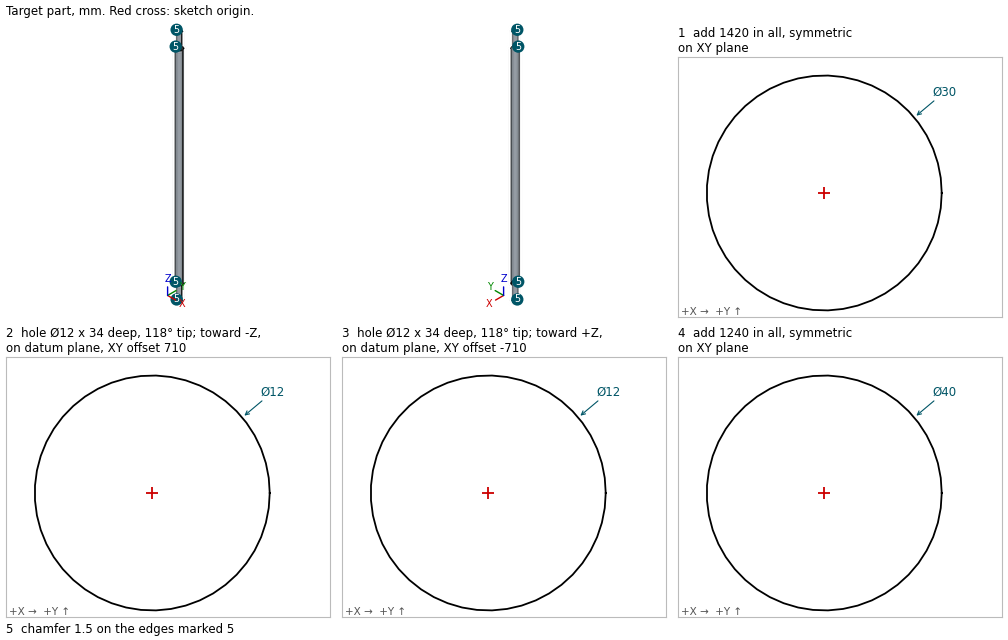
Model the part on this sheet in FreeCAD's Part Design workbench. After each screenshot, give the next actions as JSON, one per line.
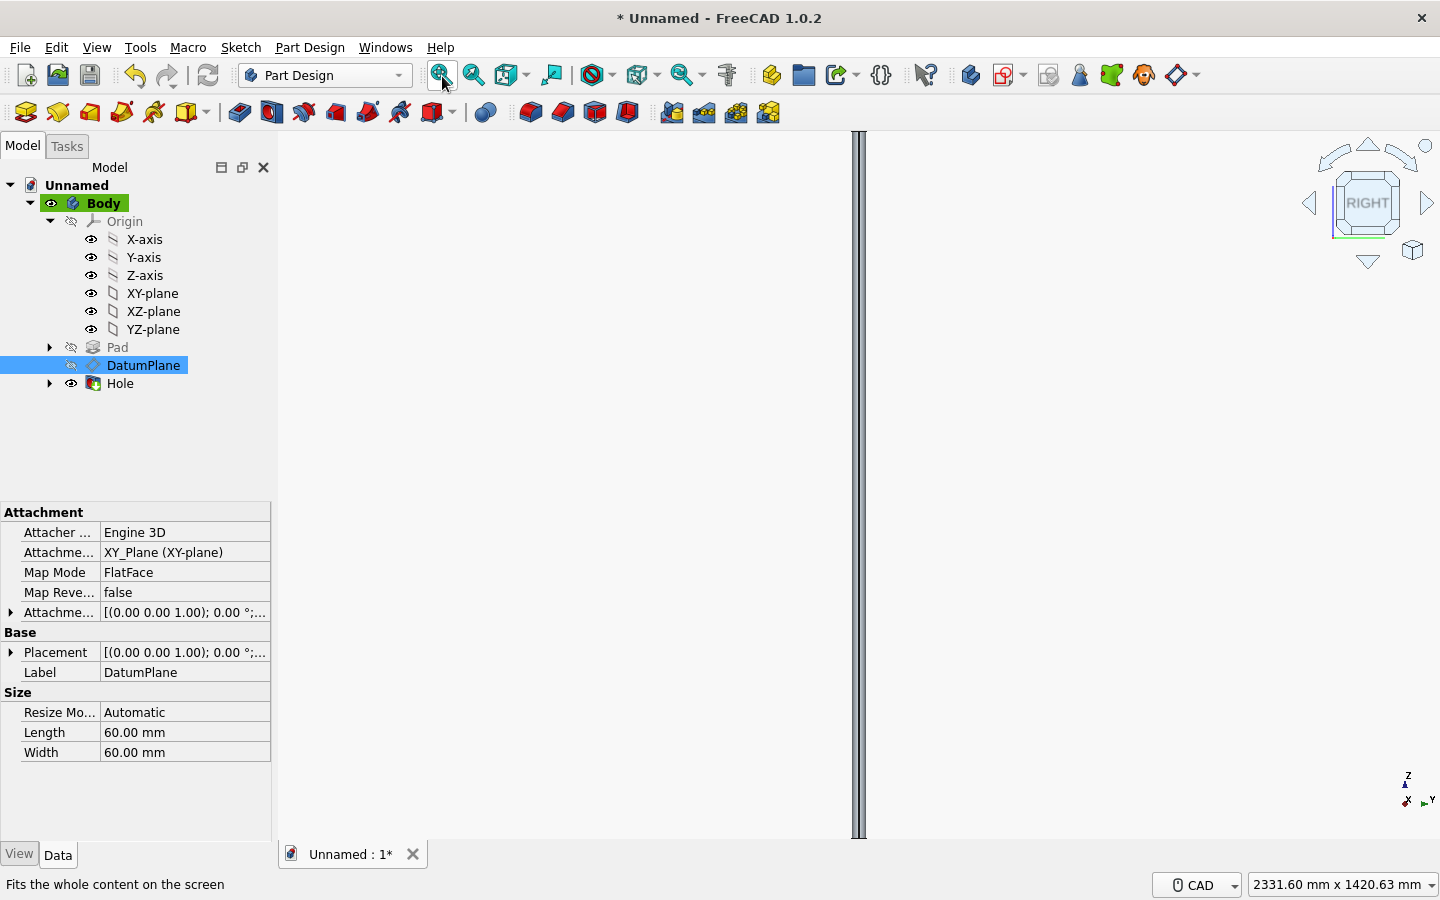
{"action": "left_click", "coordinate": [136, 293]}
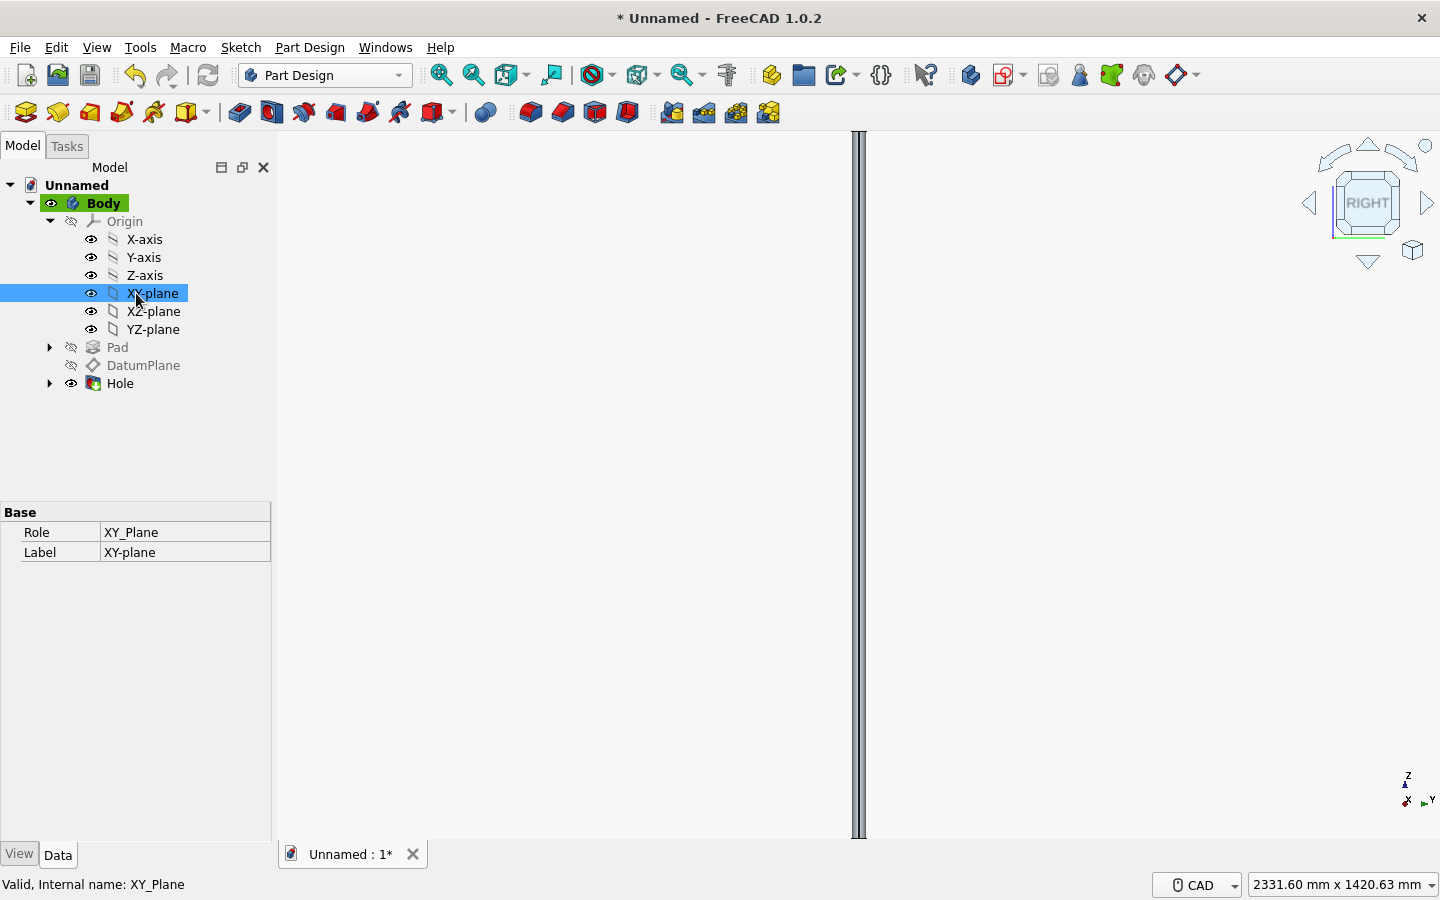
{"action": "left_click", "coordinate": [1176, 76]}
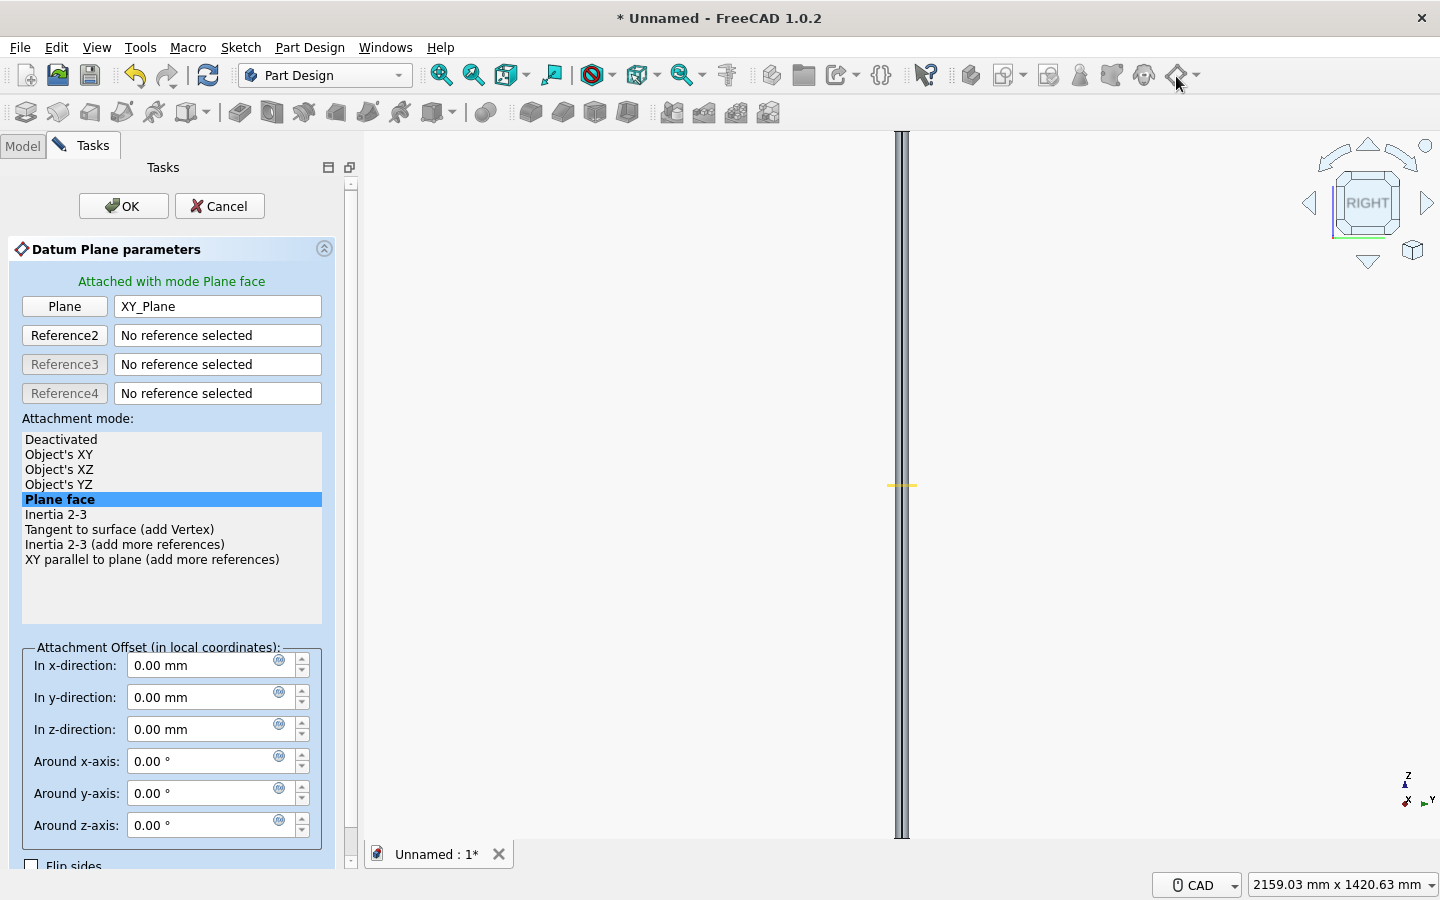
{"action": "triple_click", "coordinate": [210, 729]}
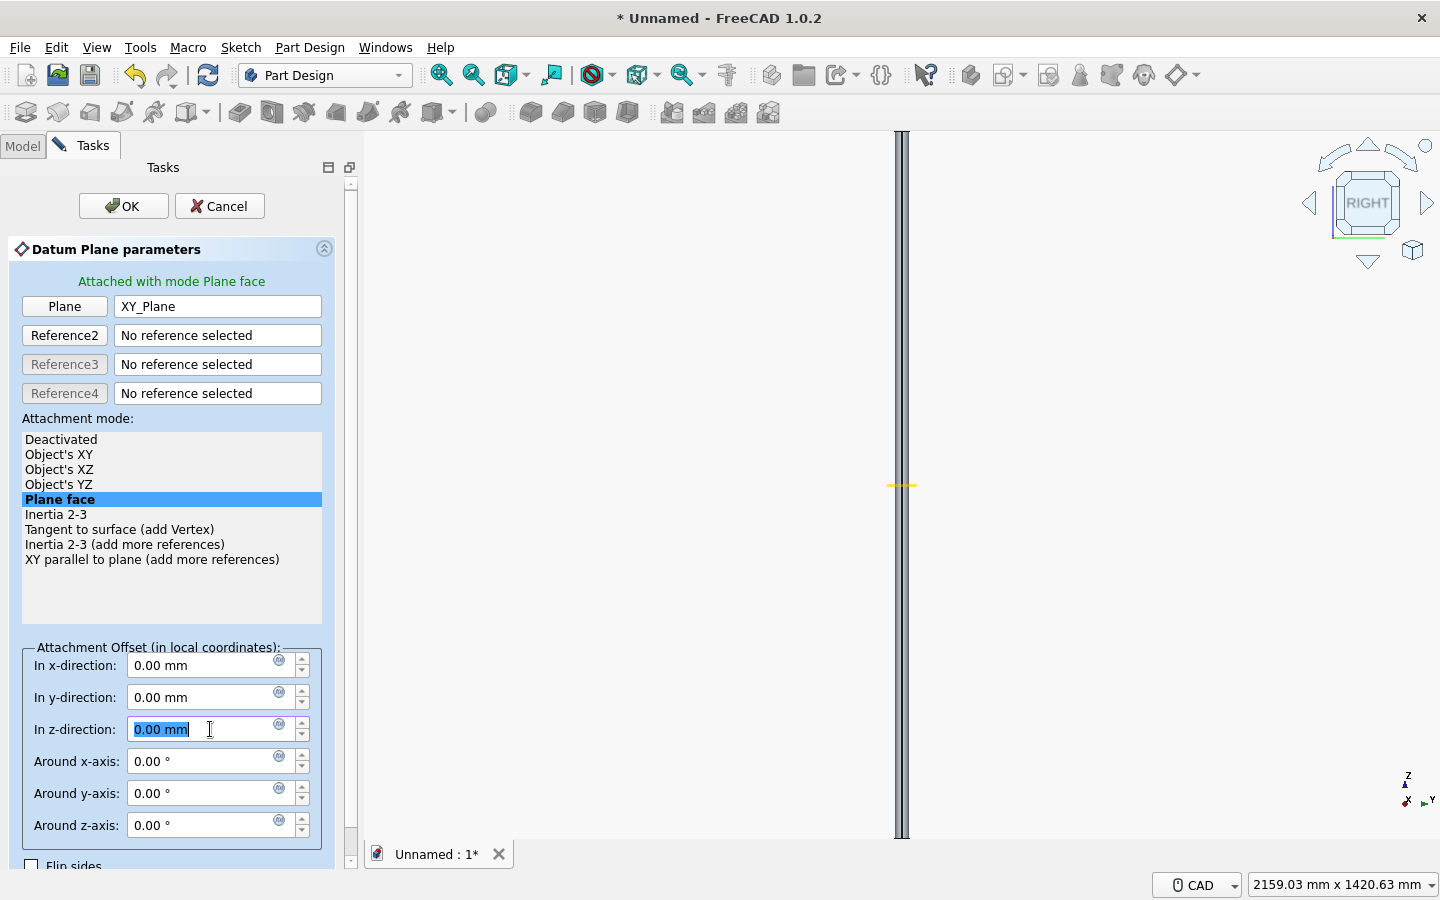
{"action": "type", "text": "-710"}
{"action": "key", "text": "Tab"}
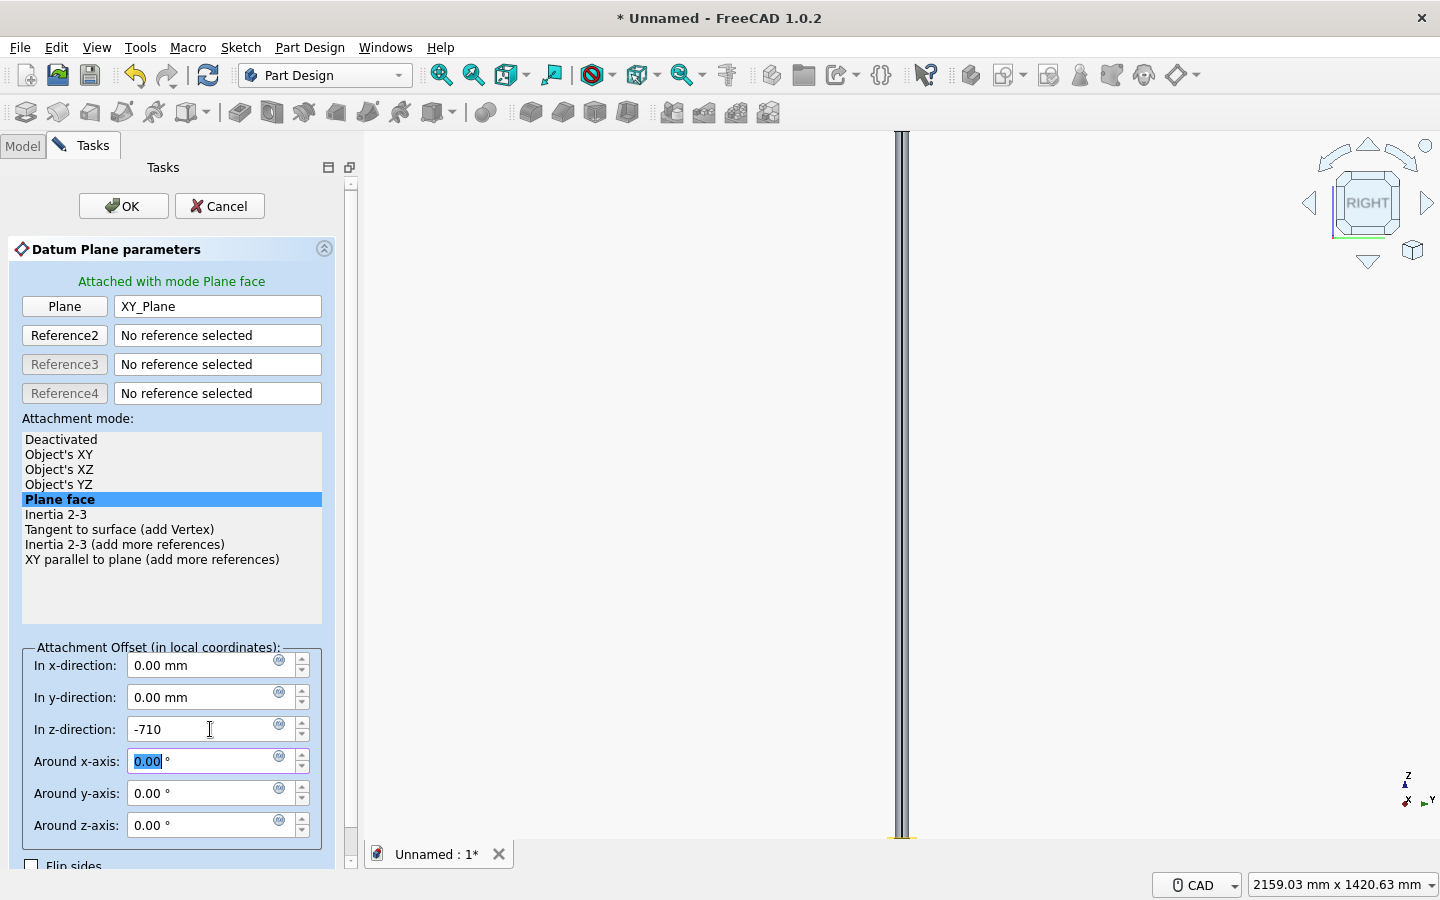
{"action": "left_click", "coordinate": [124, 206]}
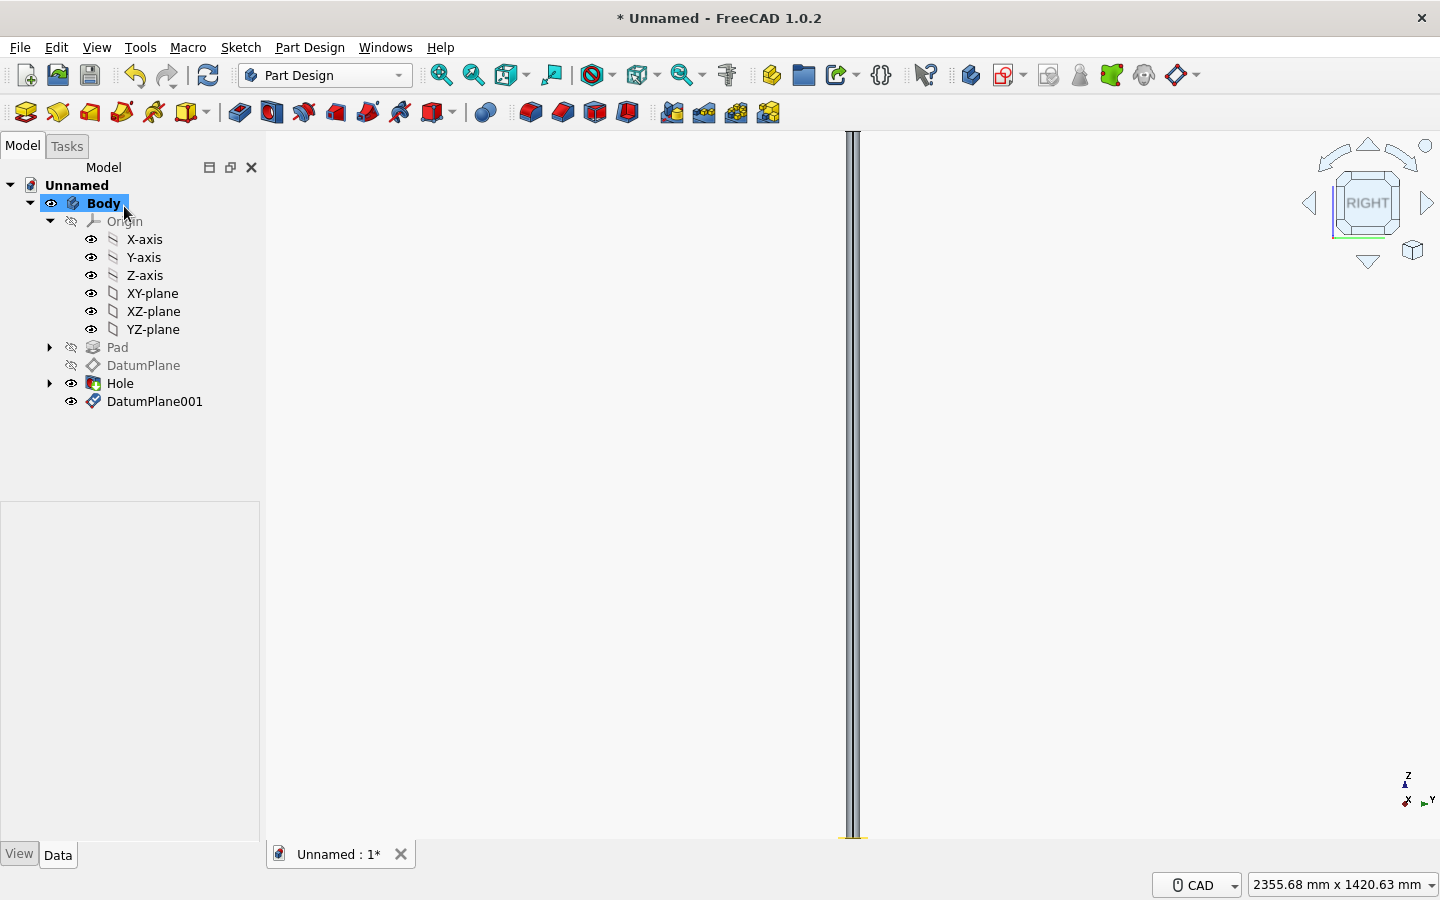
{"action": "left_click", "coordinate": [116, 401]}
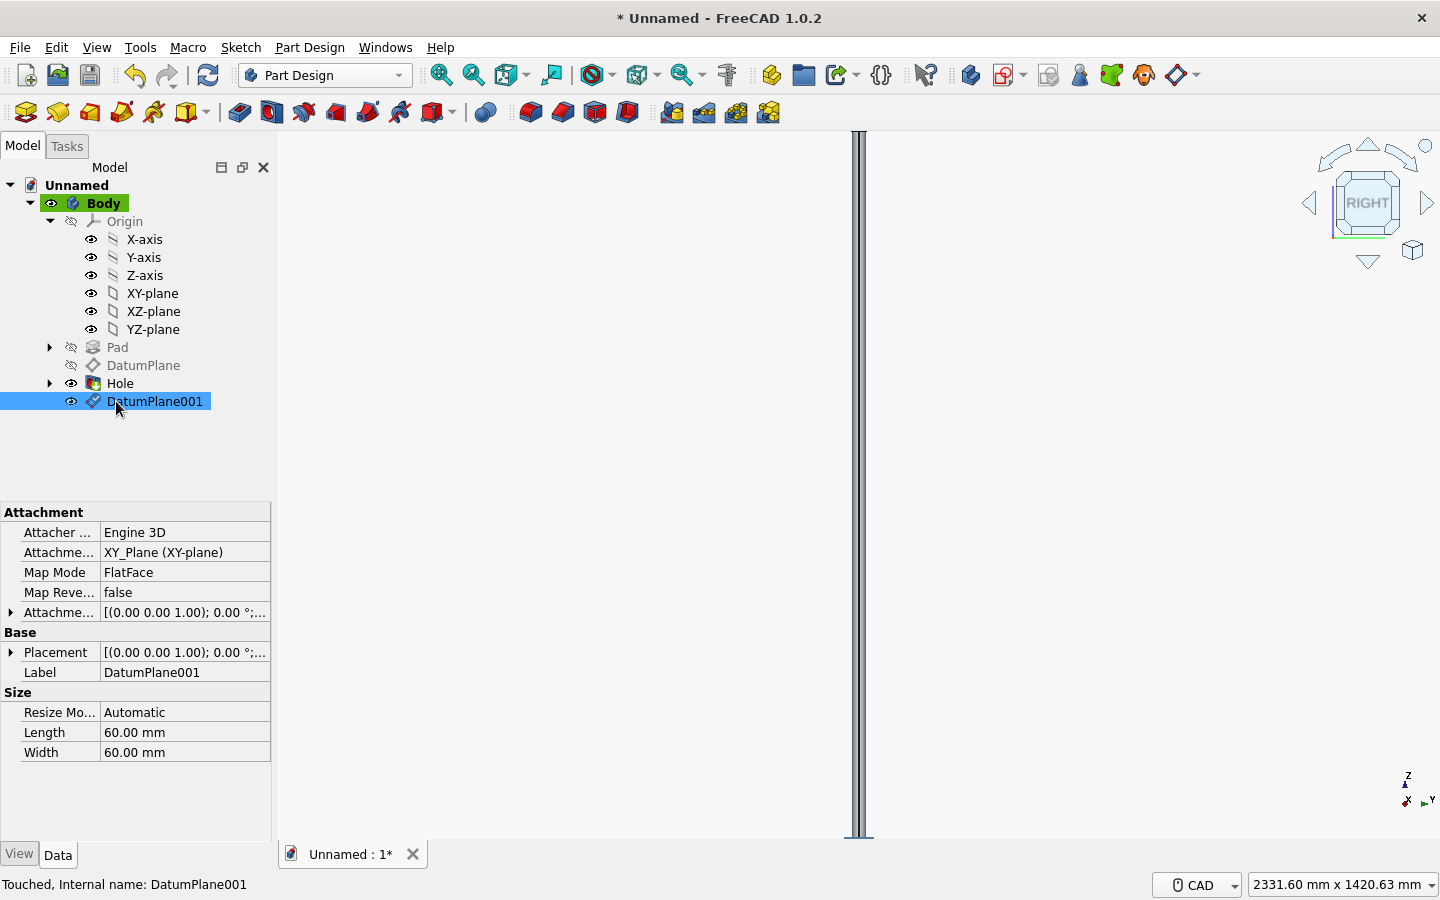
{"action": "left_click", "coordinate": [1004, 76]}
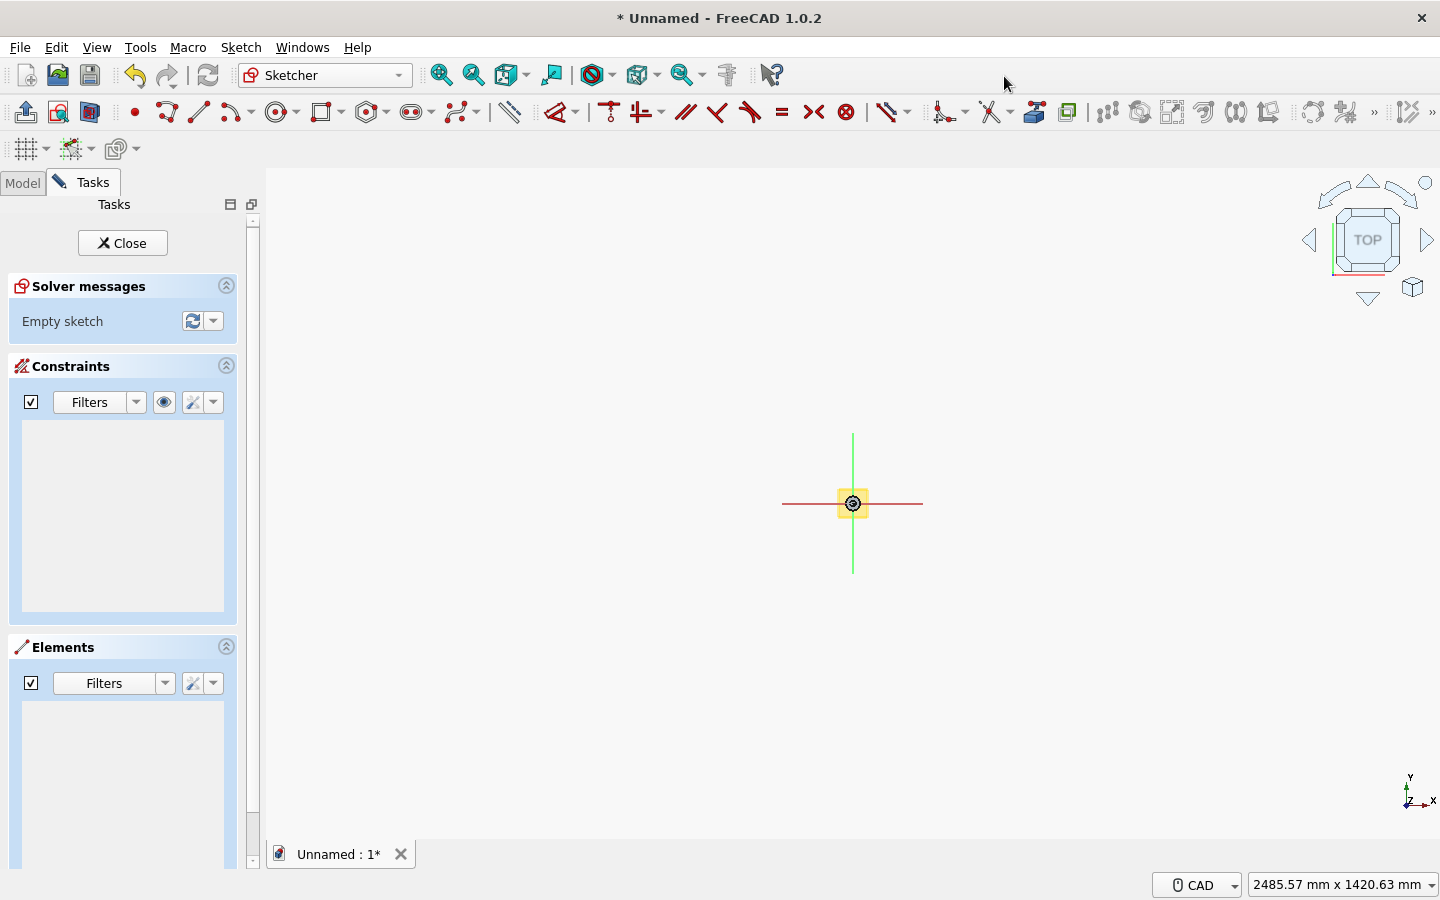
{"action": "left_click", "coordinate": [90, 112]}